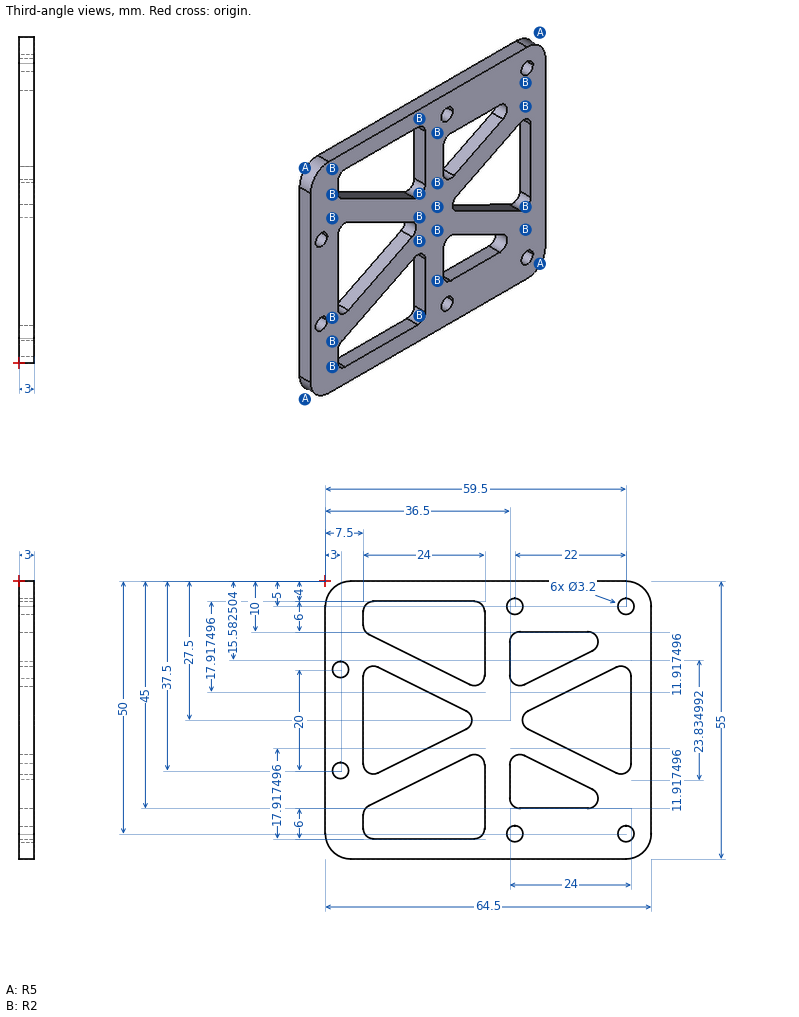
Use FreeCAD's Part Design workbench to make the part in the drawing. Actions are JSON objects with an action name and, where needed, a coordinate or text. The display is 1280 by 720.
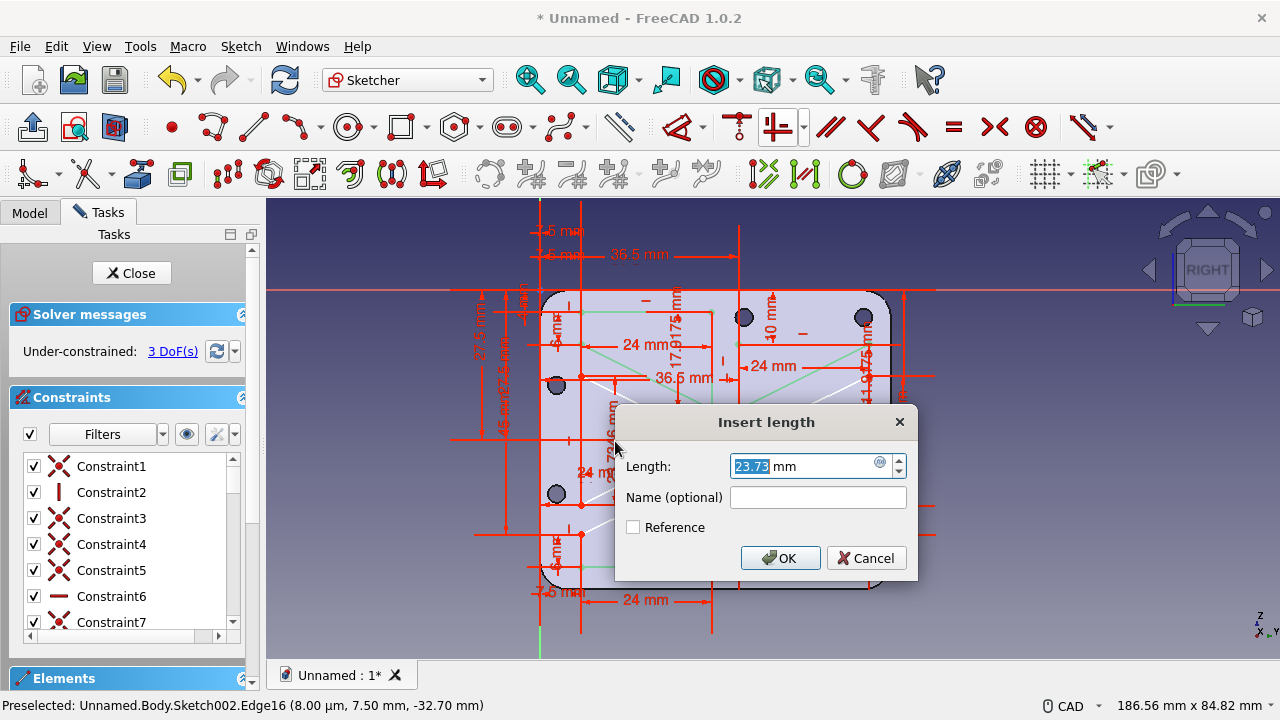
{"action": "type", "text": "23.834992"}
{"action": "key", "text": "Return"}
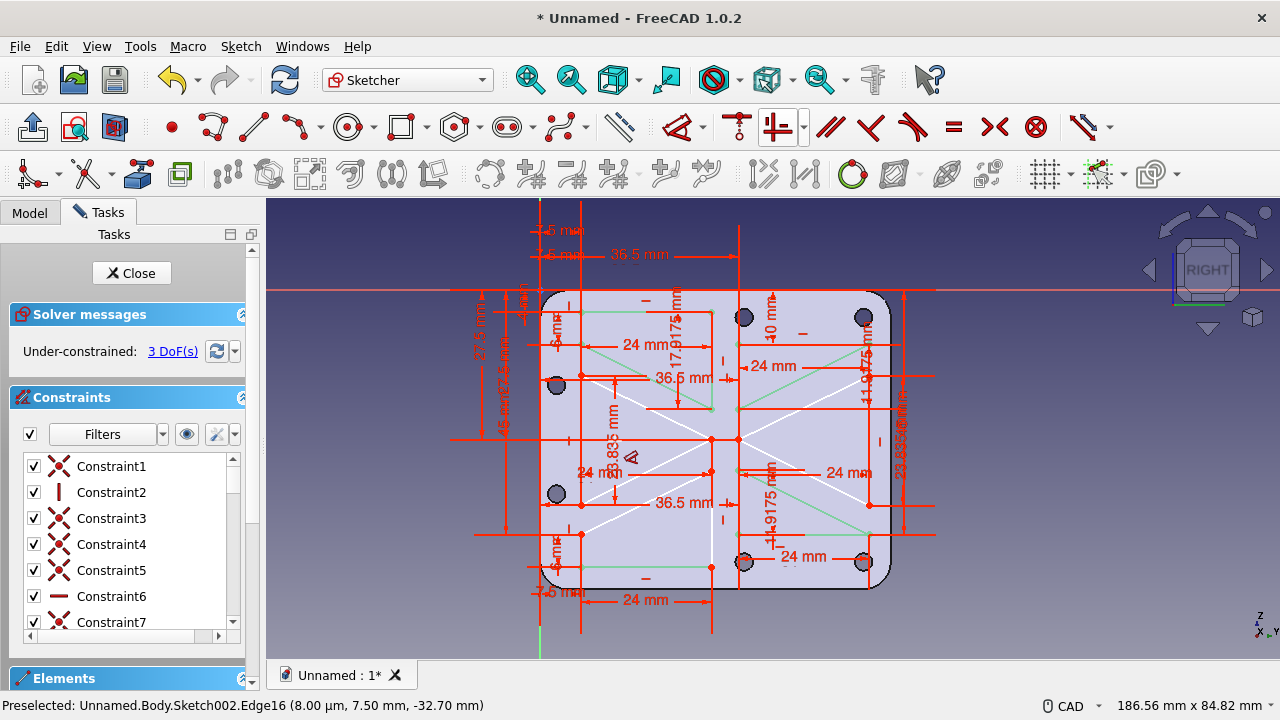
{"action": "left_click", "coordinate": [712, 500]}
{"action": "left_click", "coordinate": [678, 541]}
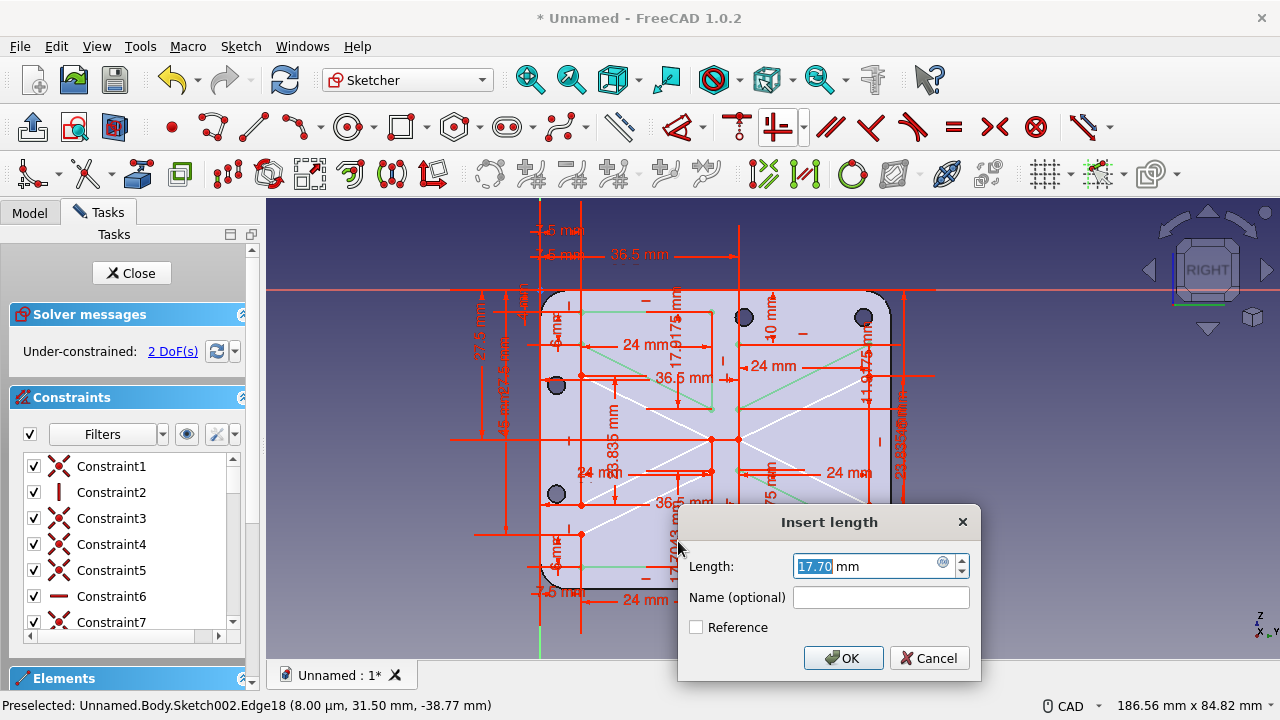
{"action": "type", "text": "17.917496"}
{"action": "key", "text": "Return"}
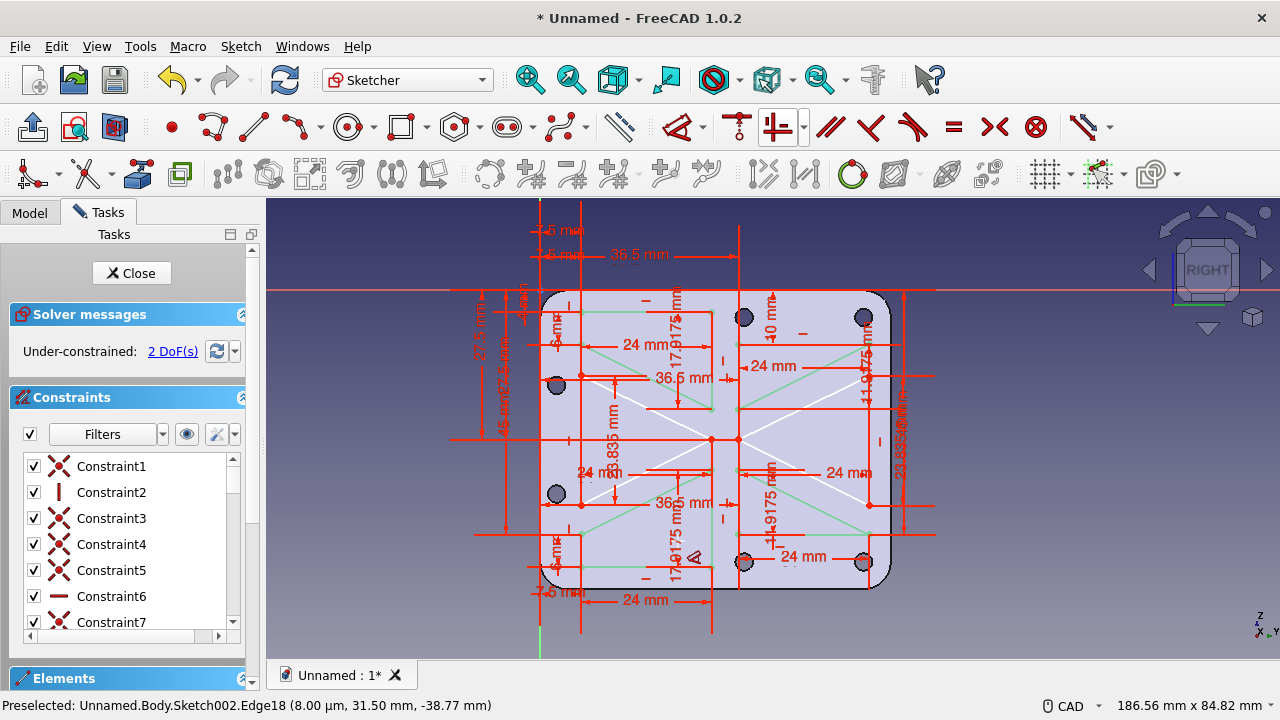
{"action": "left_click", "coordinate": [869, 376]}
{"action": "left_click", "coordinate": [903, 333]}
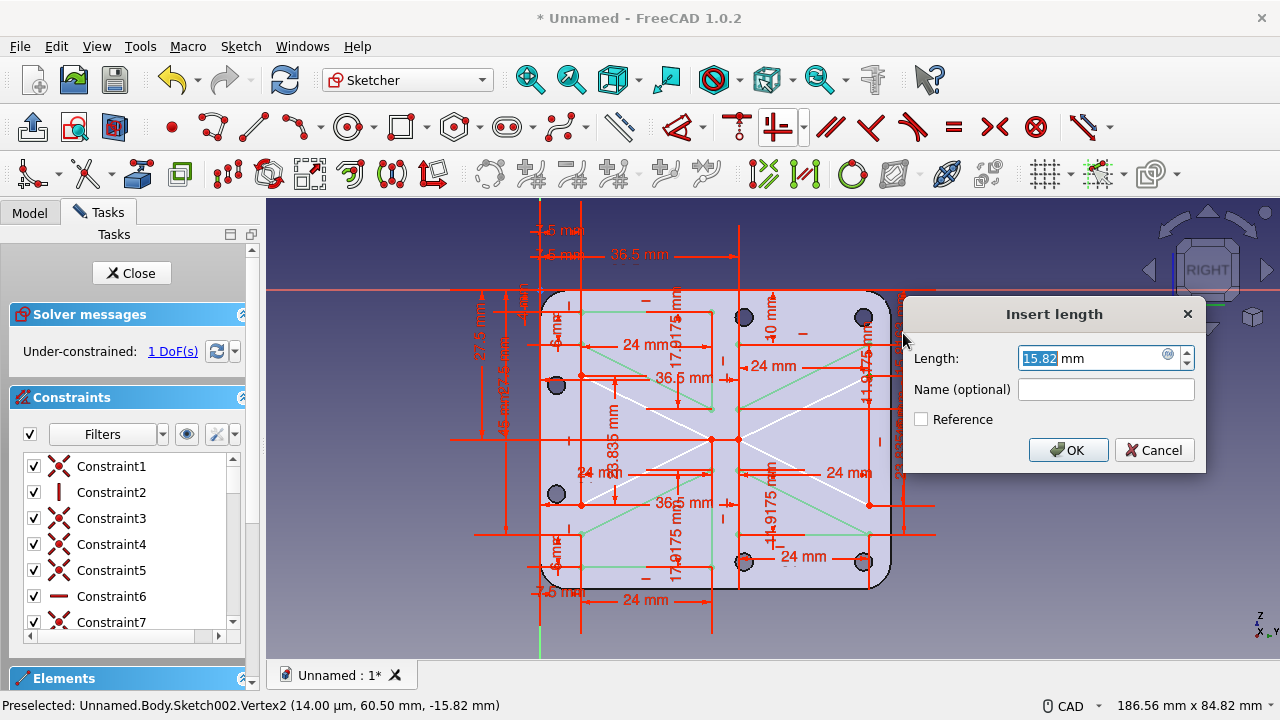
{"action": "type", "text": "15.582504"}
{"action": "key", "text": "Return"}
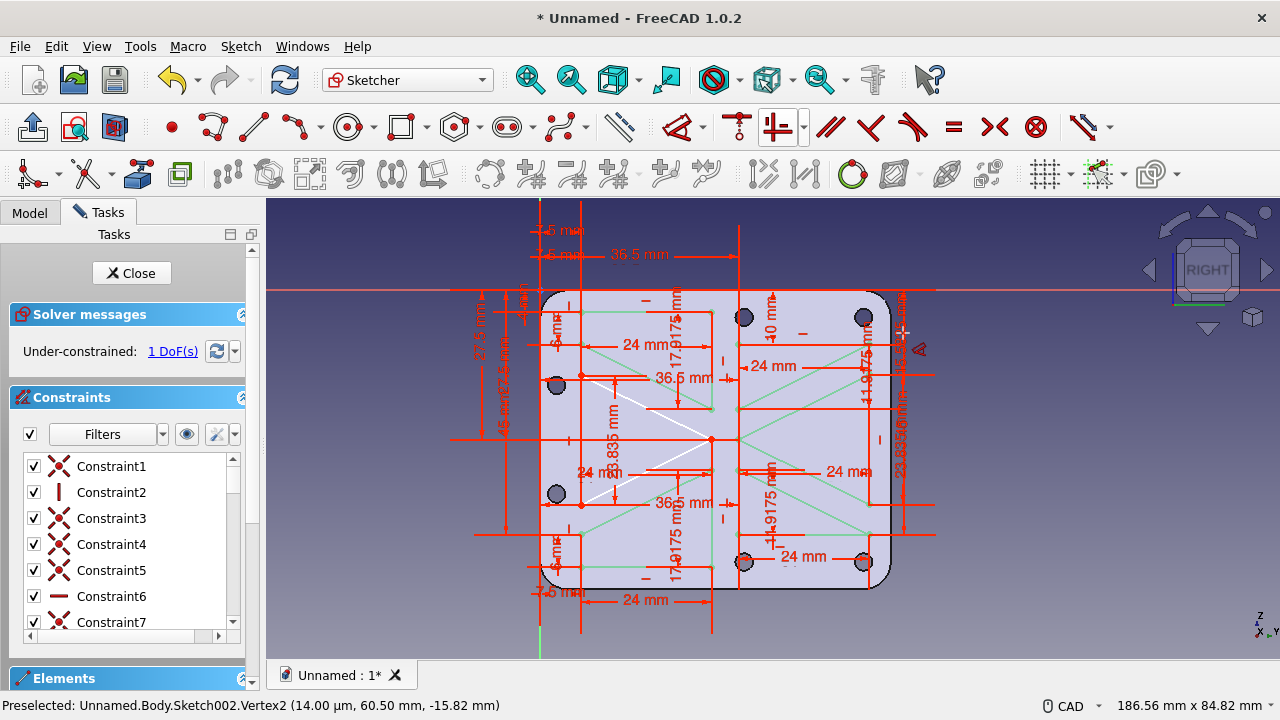
{"action": "left_click", "coordinate": [581, 376]}
{"action": "left_click", "coordinate": [434, 353]}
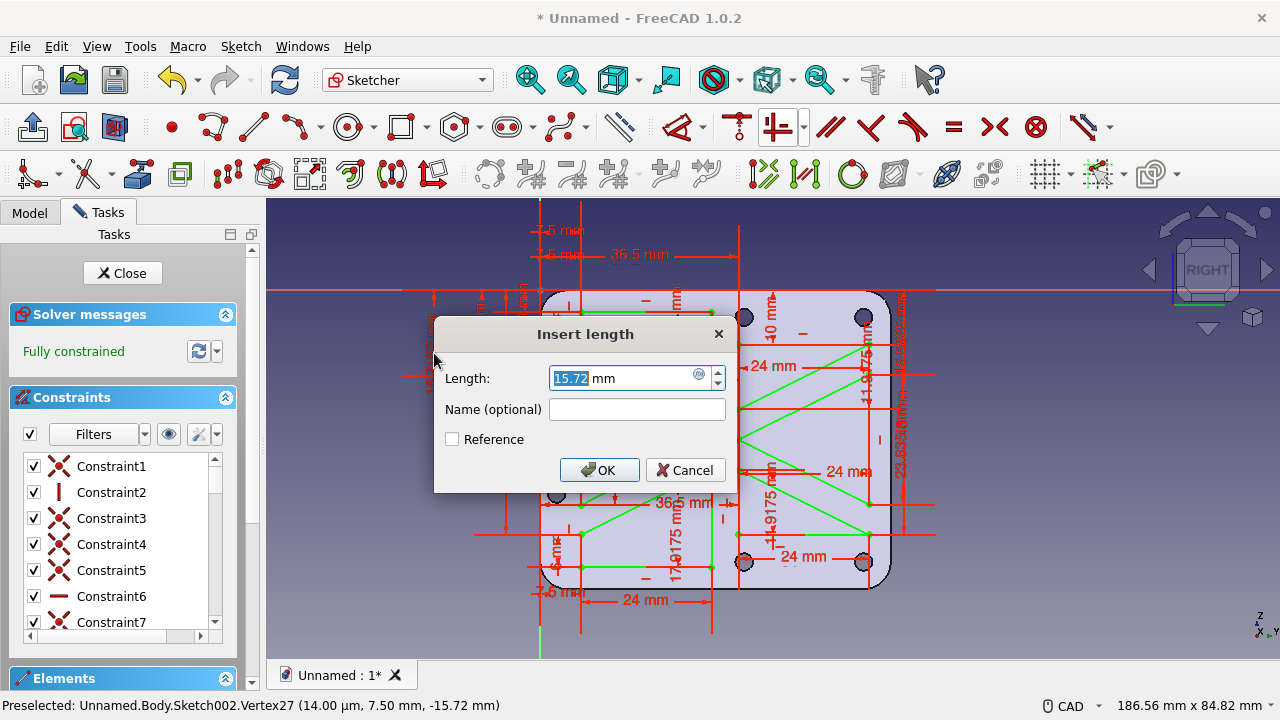
{"action": "type", "text": "15.582504"}
{"action": "key", "text": "Return"}
{"action": "key", "text": "Escape"}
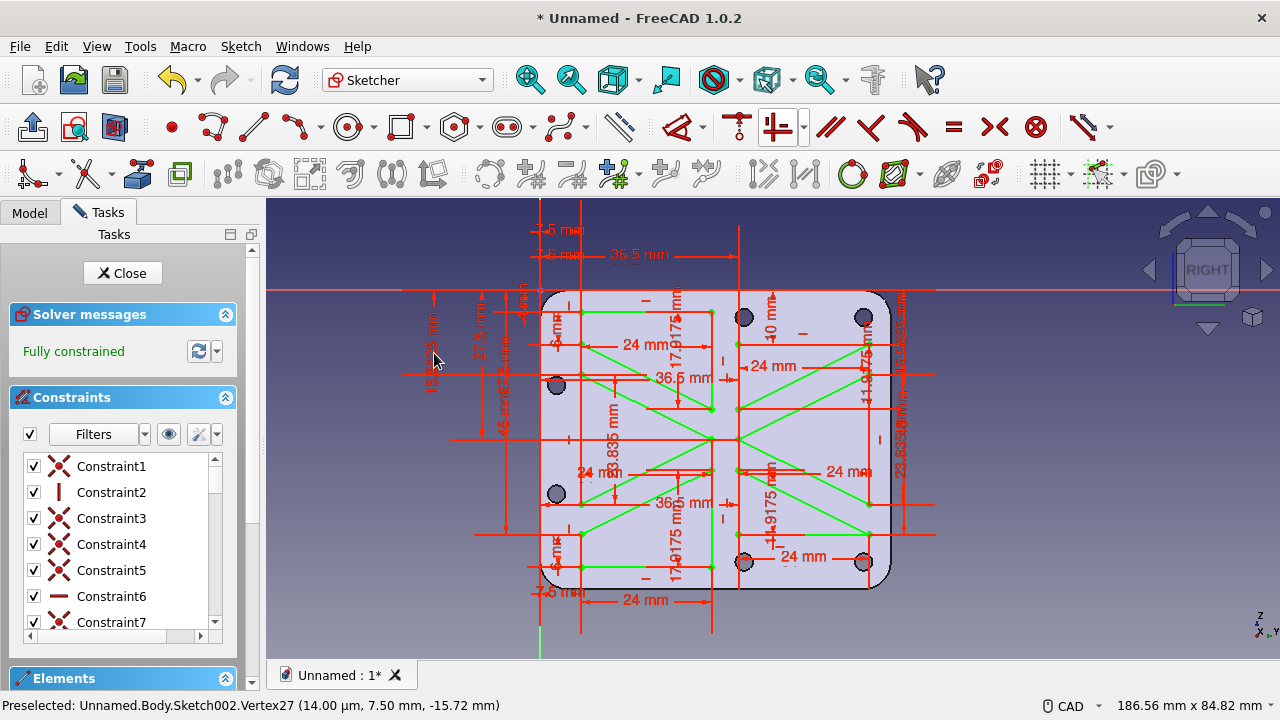
{"action": "left_click", "coordinate": [123, 273]}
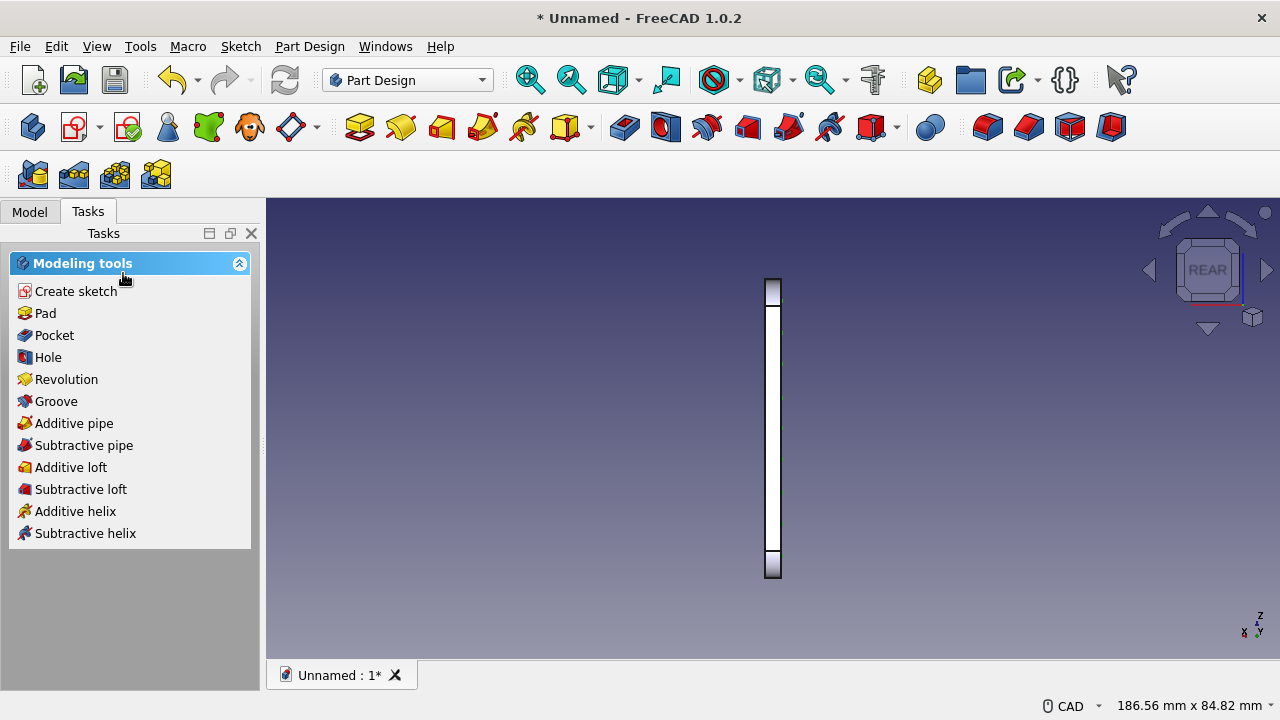
{"action": "left_click", "coordinate": [625, 128]}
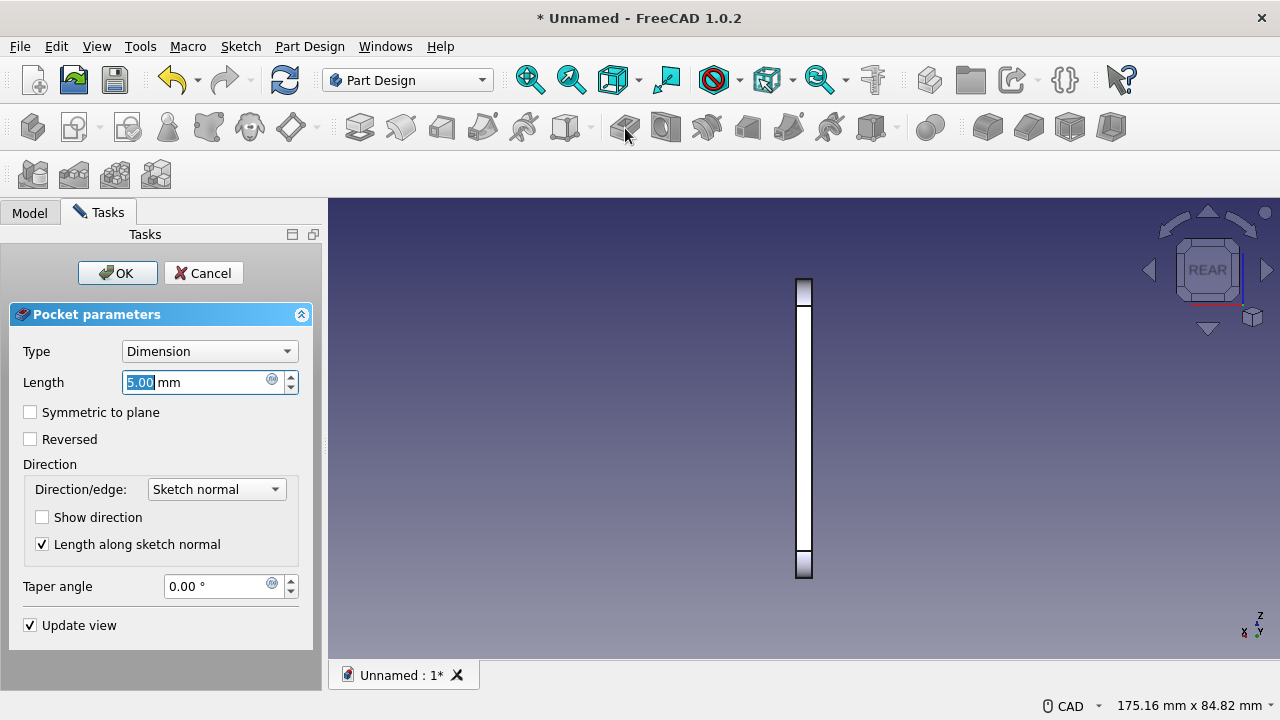
{"action": "type", "text": "3"}
{"action": "key", "text": "Tab"}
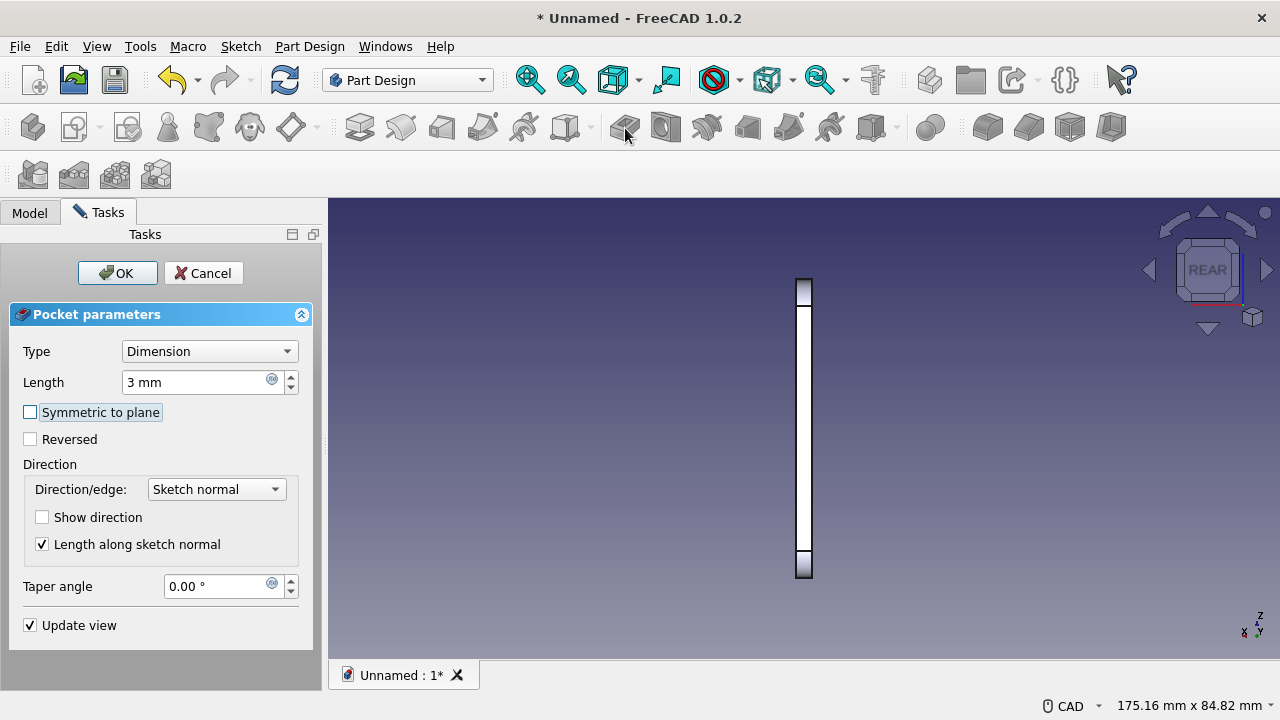
{"action": "left_click", "coordinate": [31, 439]}